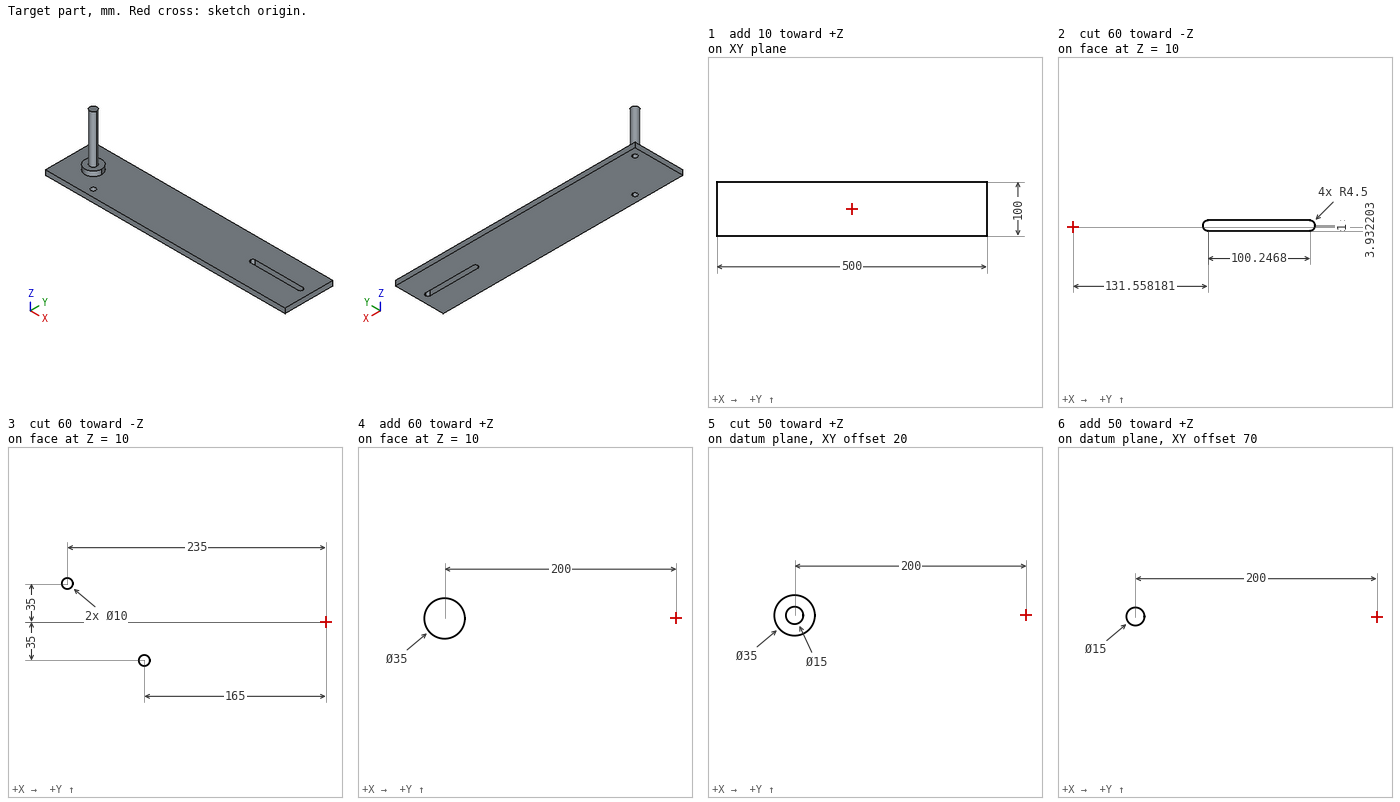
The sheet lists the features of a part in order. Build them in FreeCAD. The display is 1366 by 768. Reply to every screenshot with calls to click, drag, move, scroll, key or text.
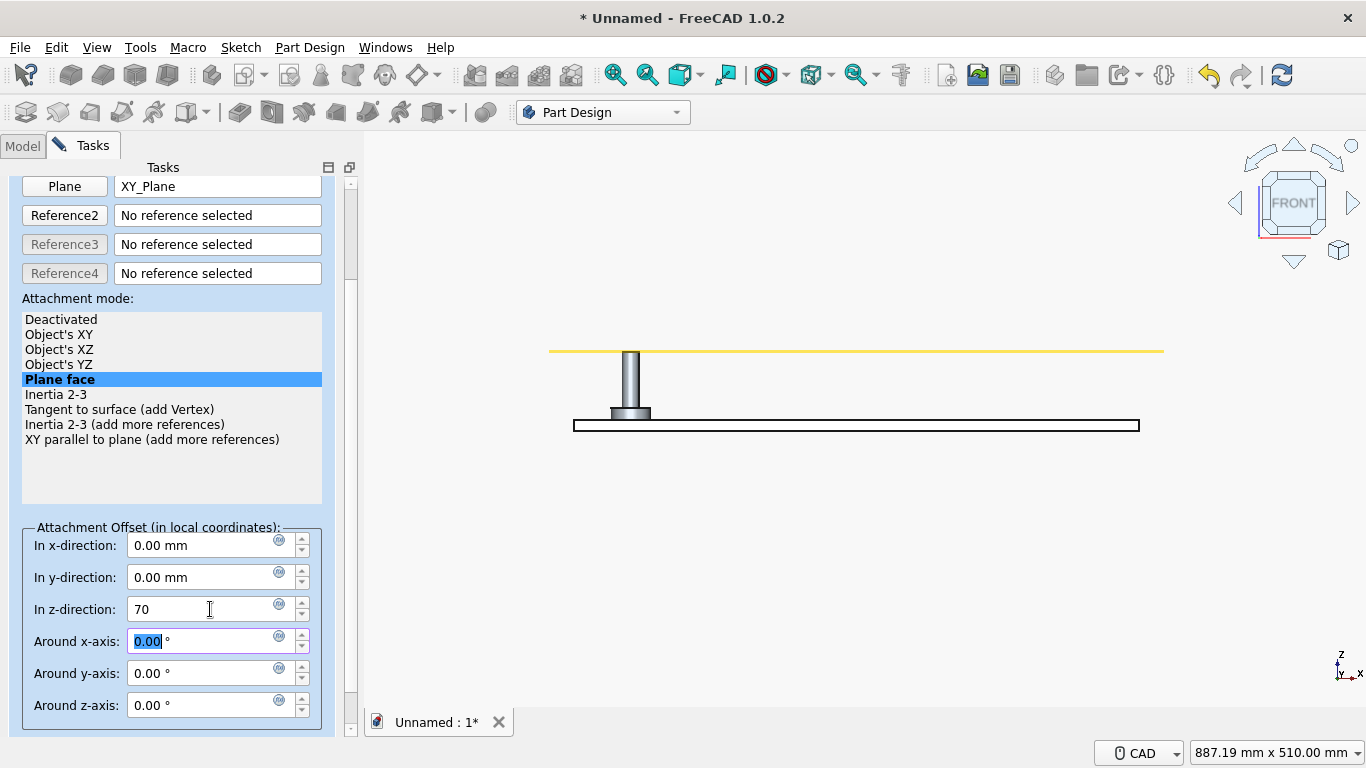
scroll(351, 456, up, 3)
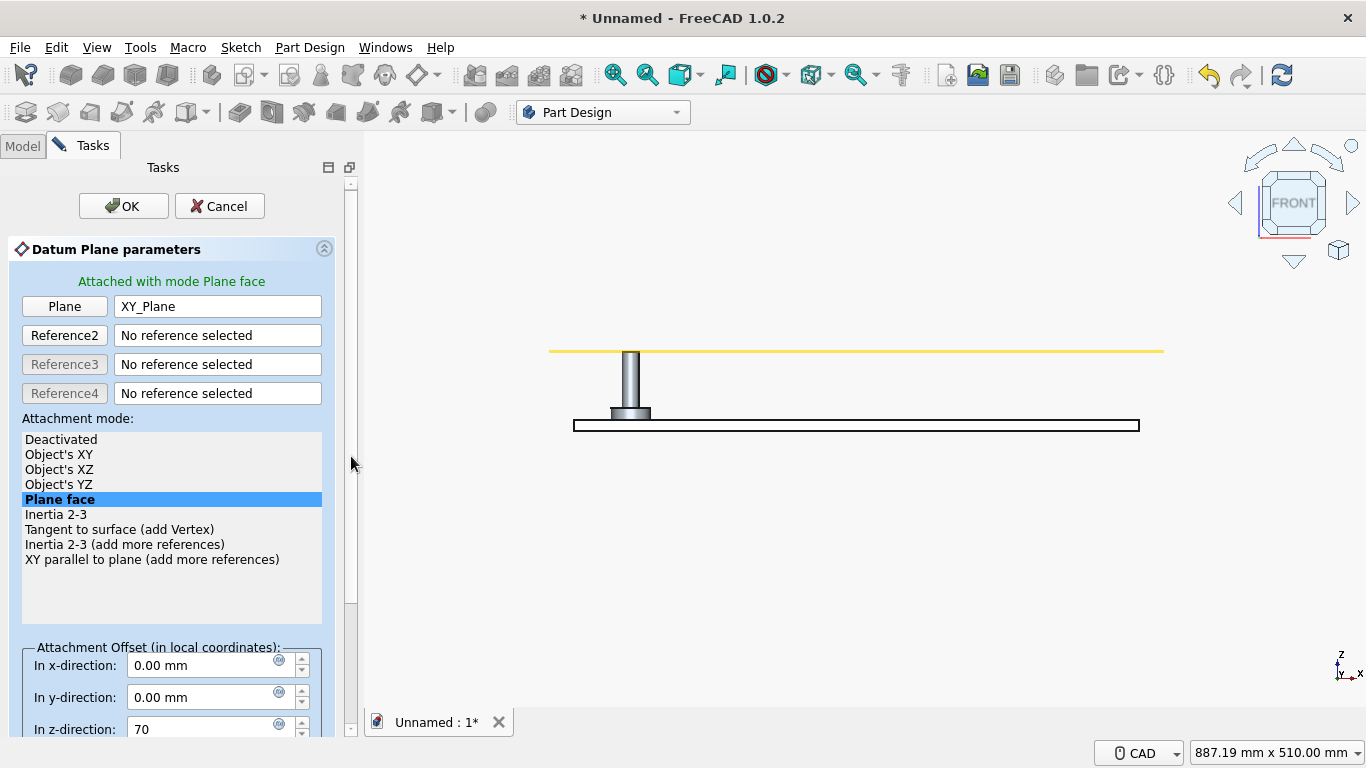
click(124, 206)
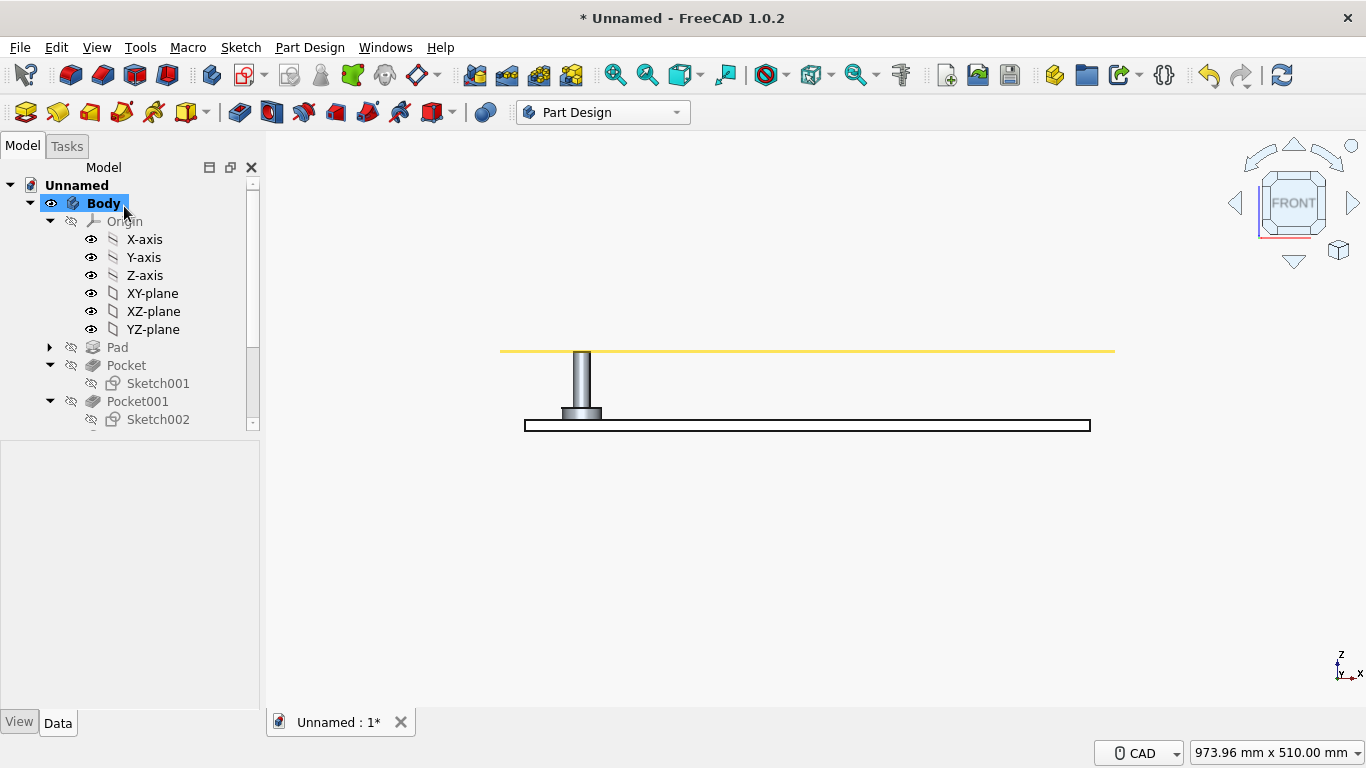
scroll(100, 307, down, 3)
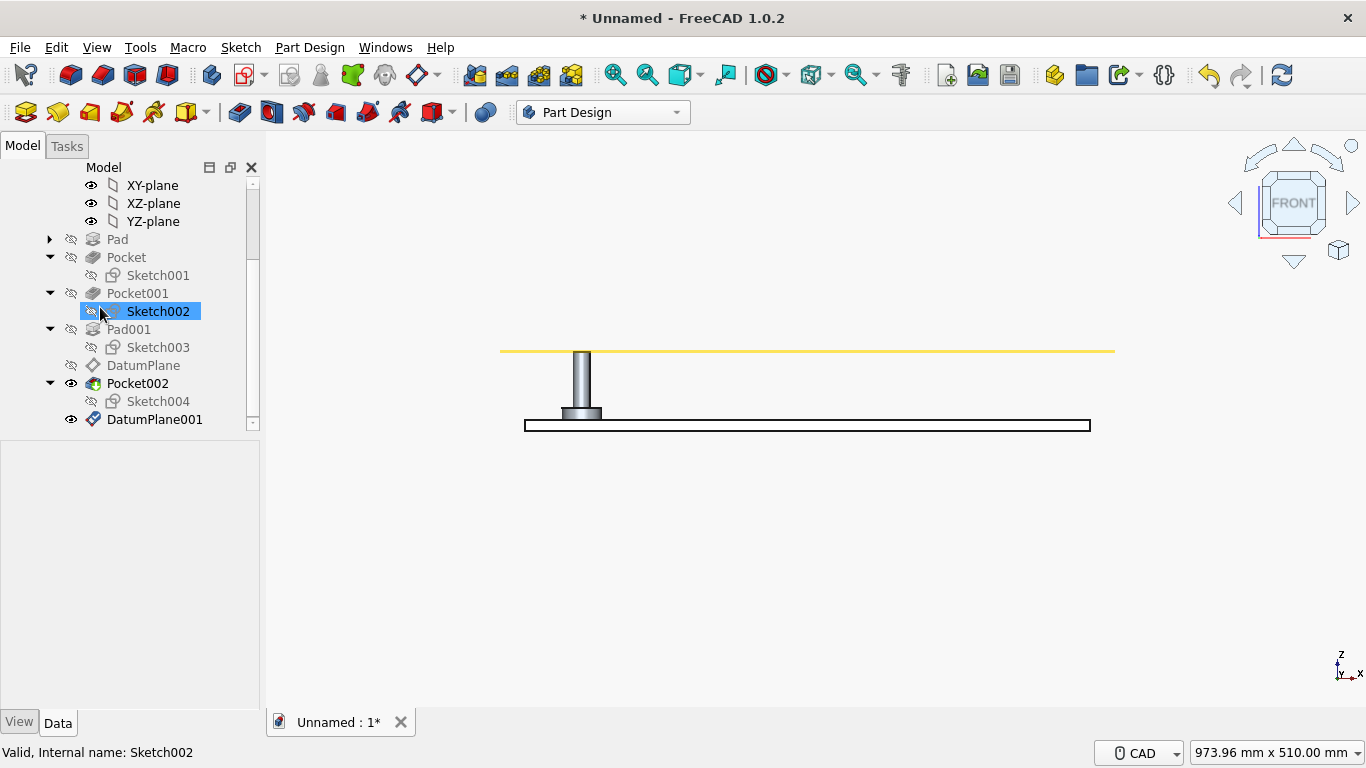
click(116, 419)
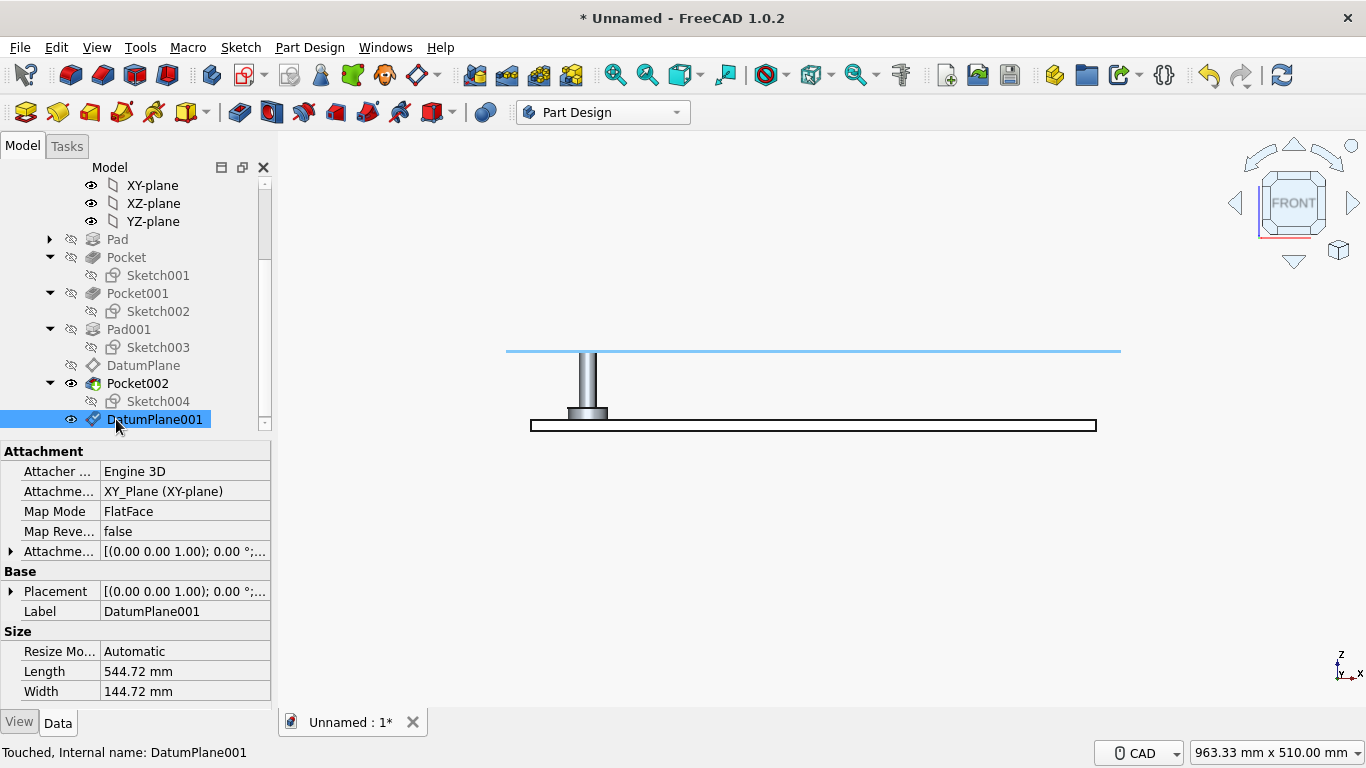
click(244, 76)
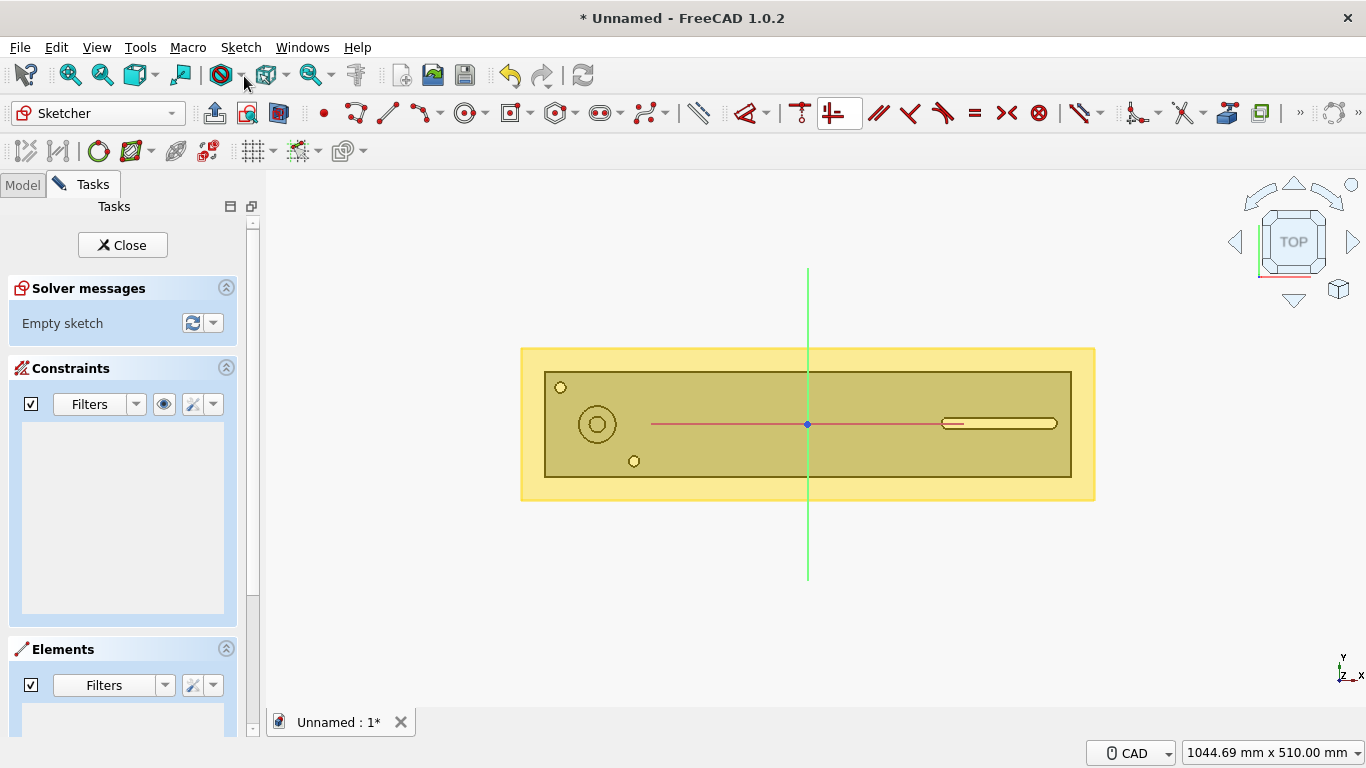
scroll(589, 424, up, 15)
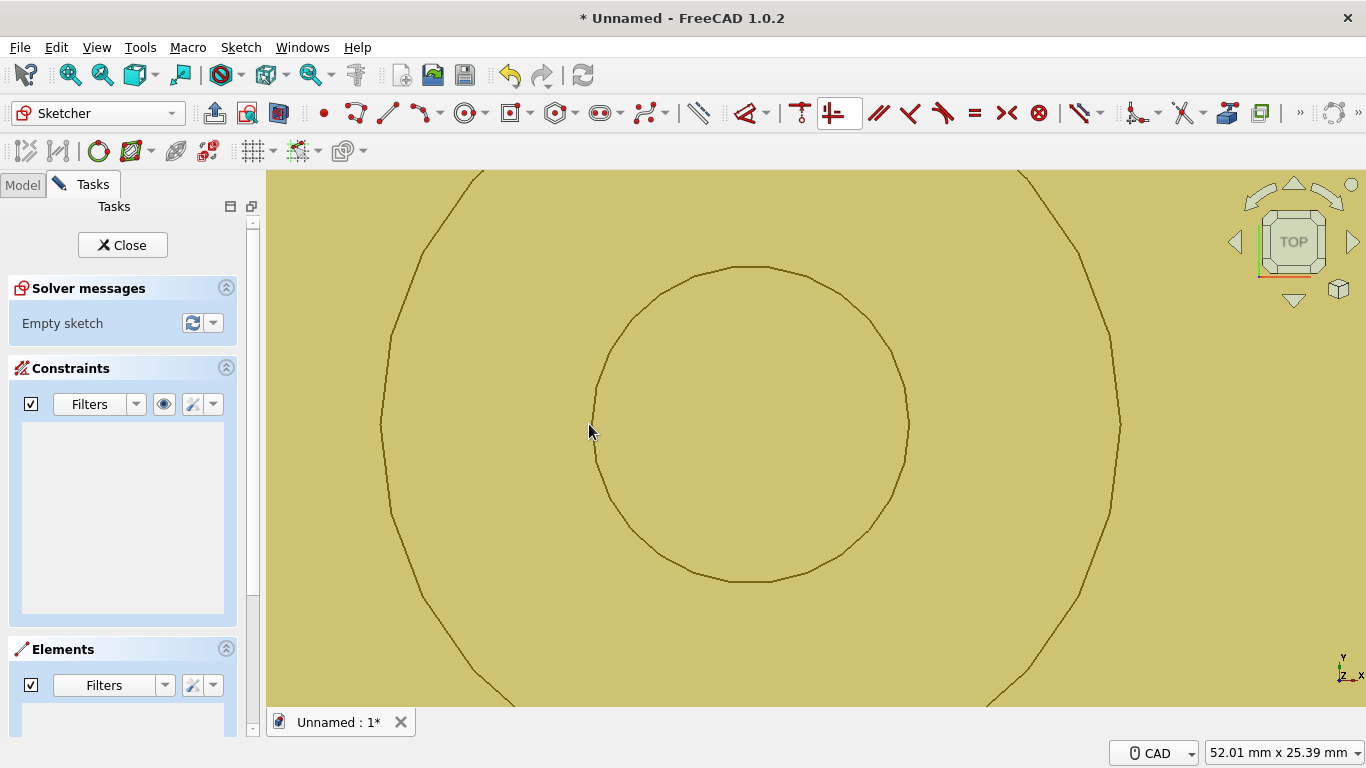
key(g)
key(c)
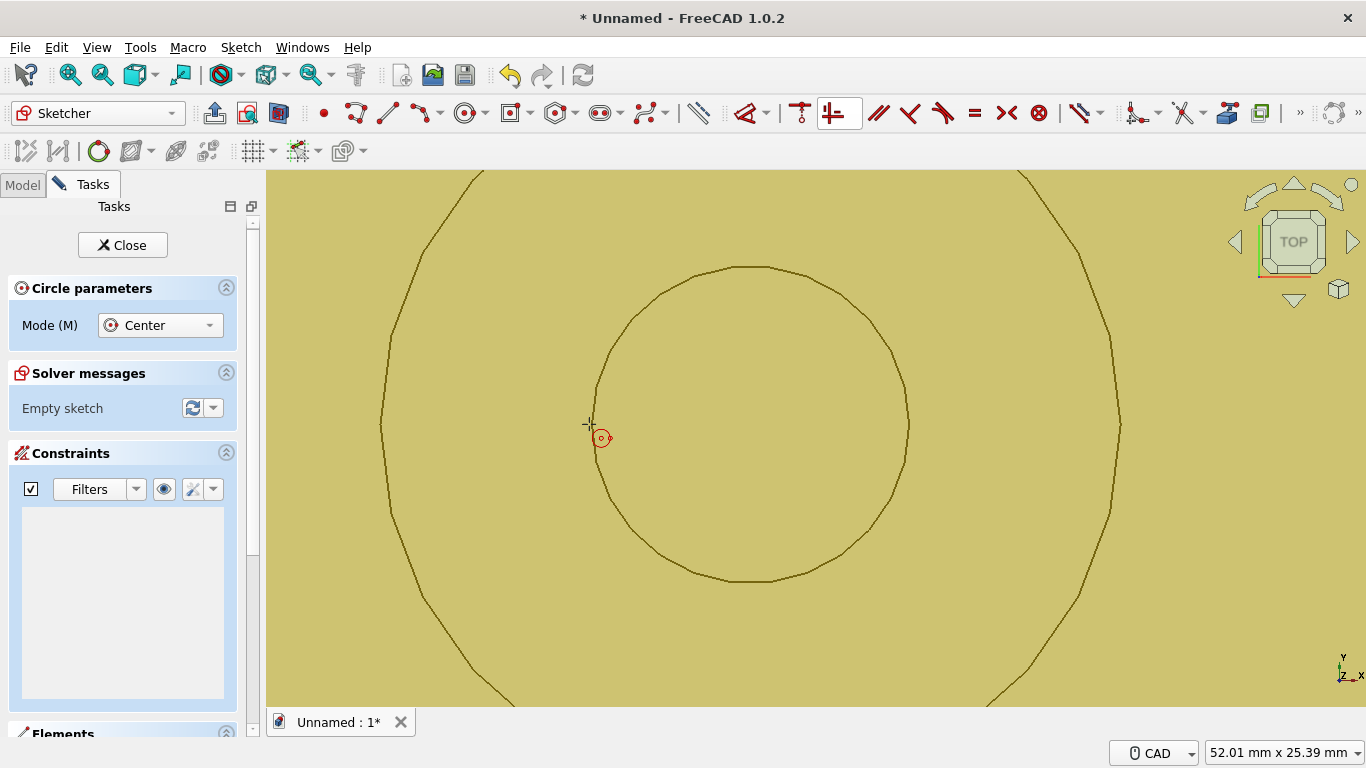
click(751, 425)
move(863, 313)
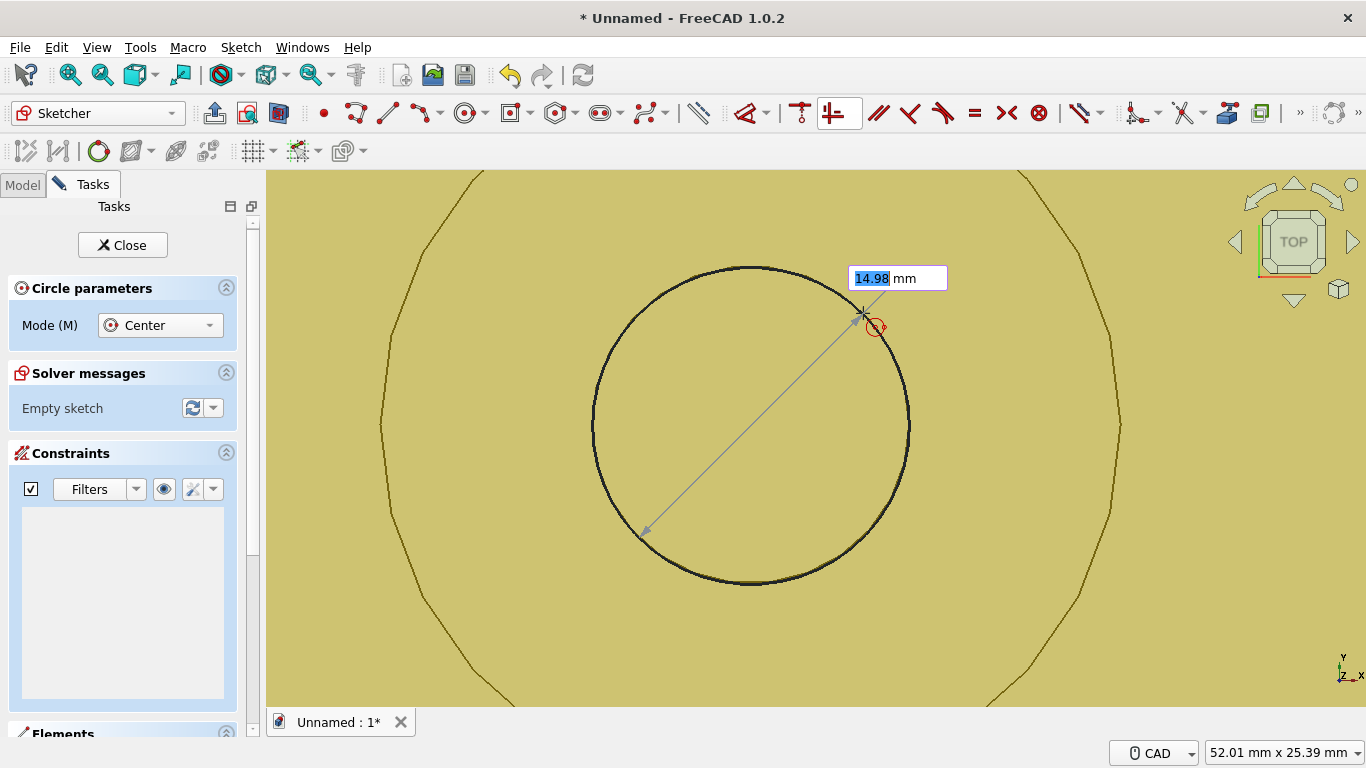
text(15)
key(Return)
key(Escape)